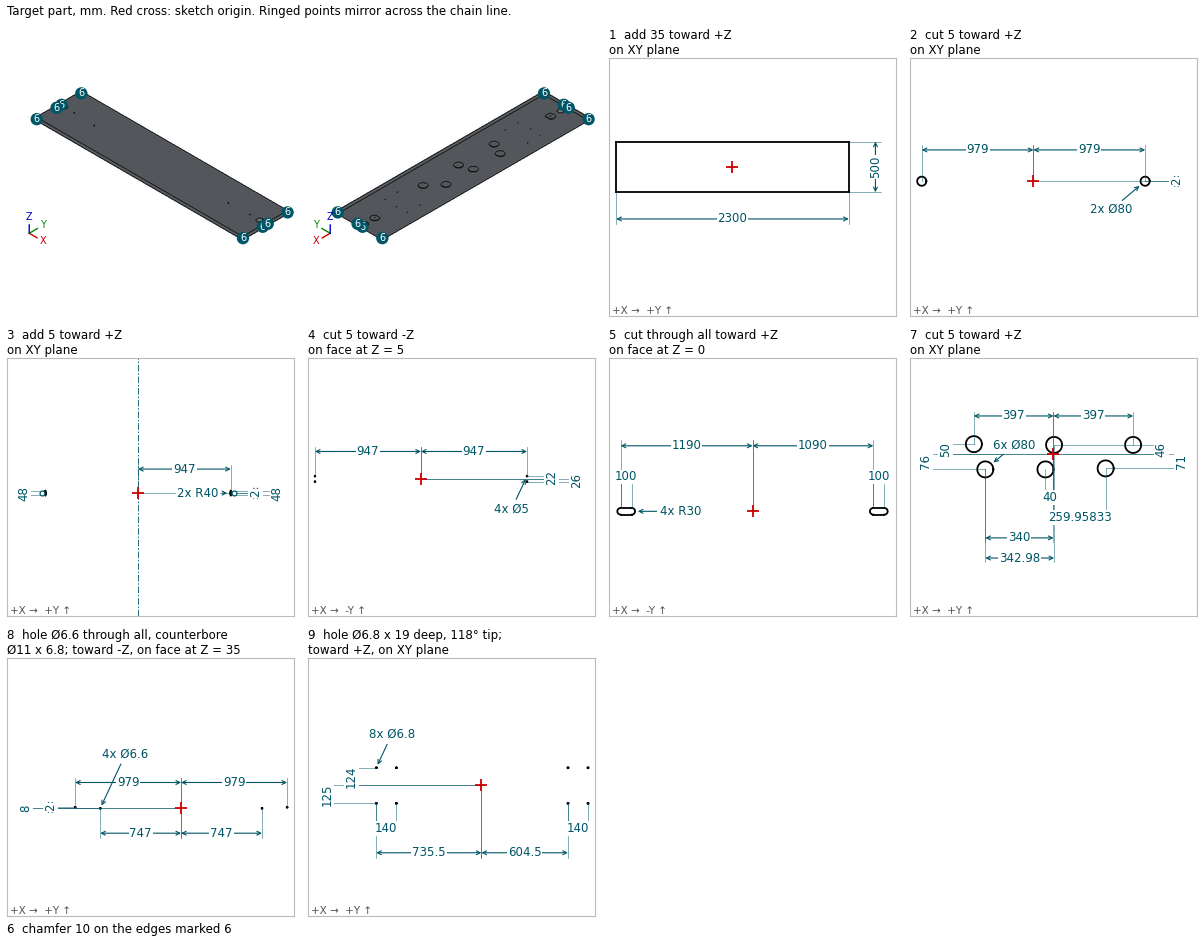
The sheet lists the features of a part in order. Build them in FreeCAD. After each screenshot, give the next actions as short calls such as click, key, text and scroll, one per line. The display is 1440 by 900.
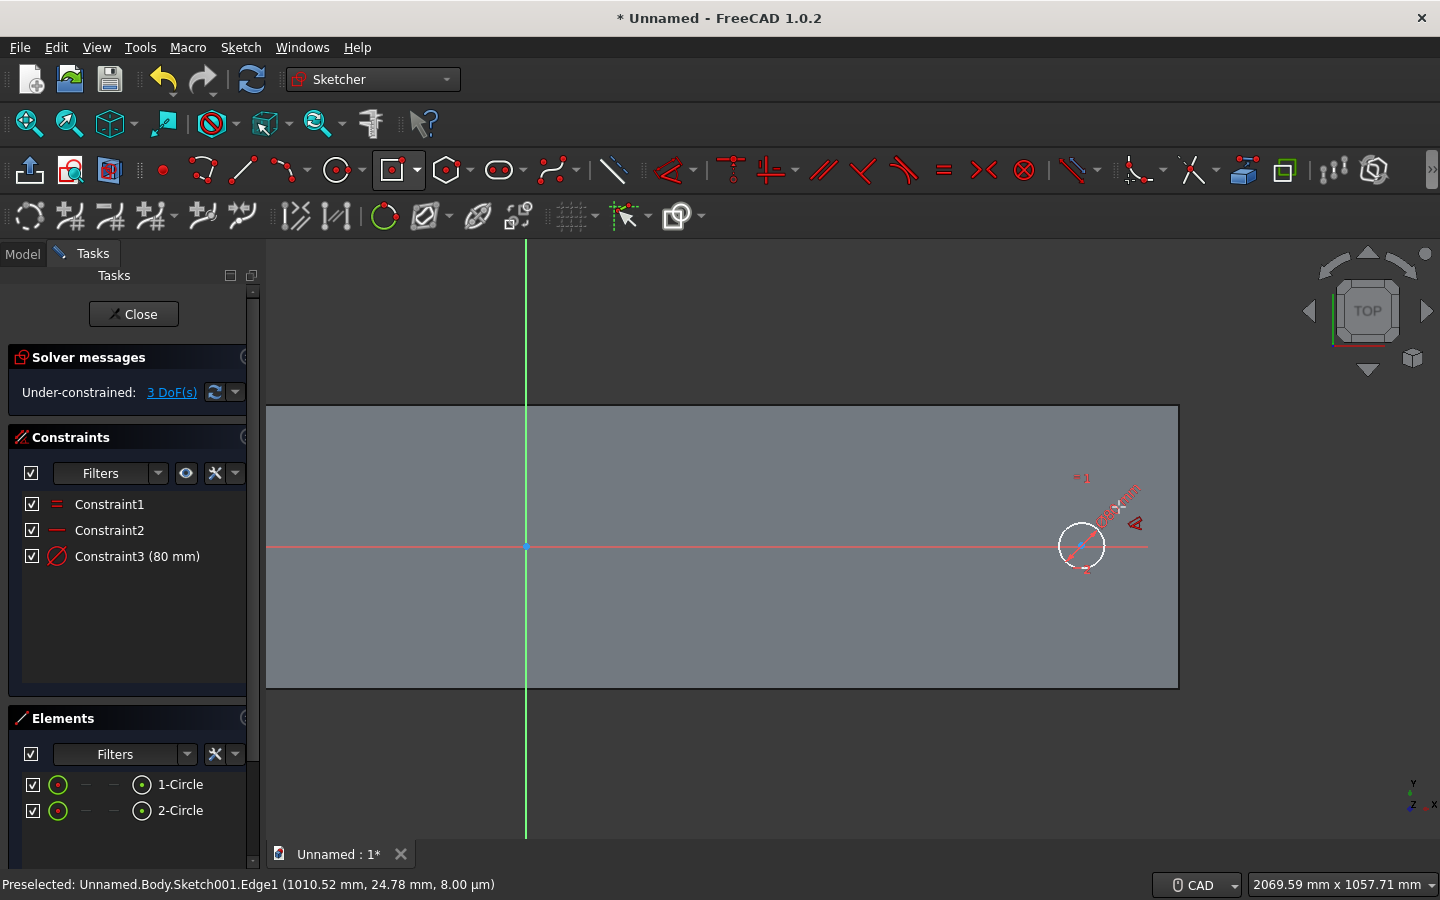
scroll(1082, 546, up, 18)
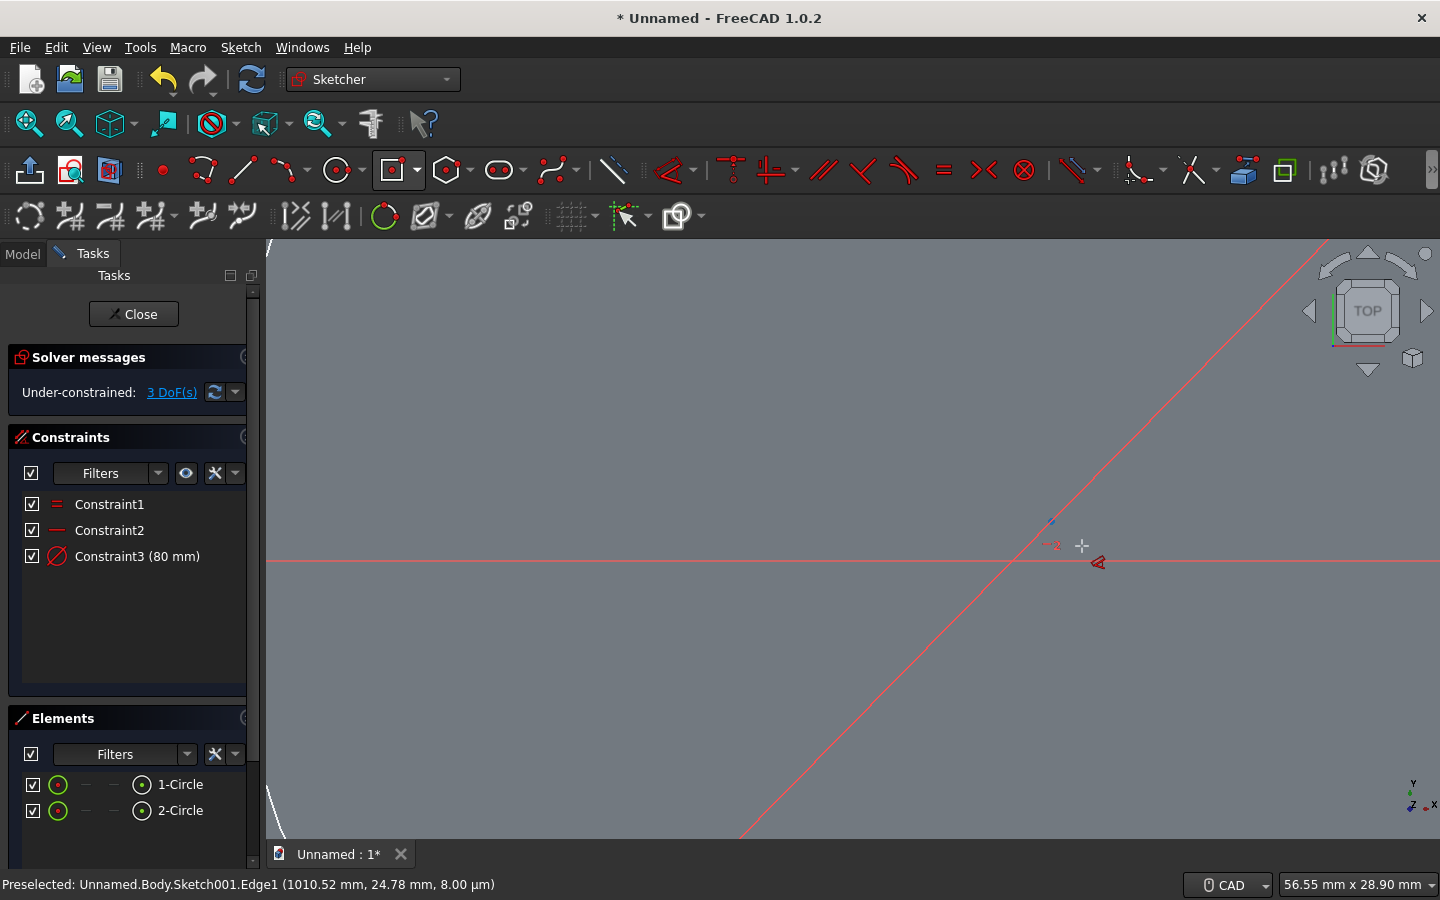
click(1052, 521)
click(1086, 541)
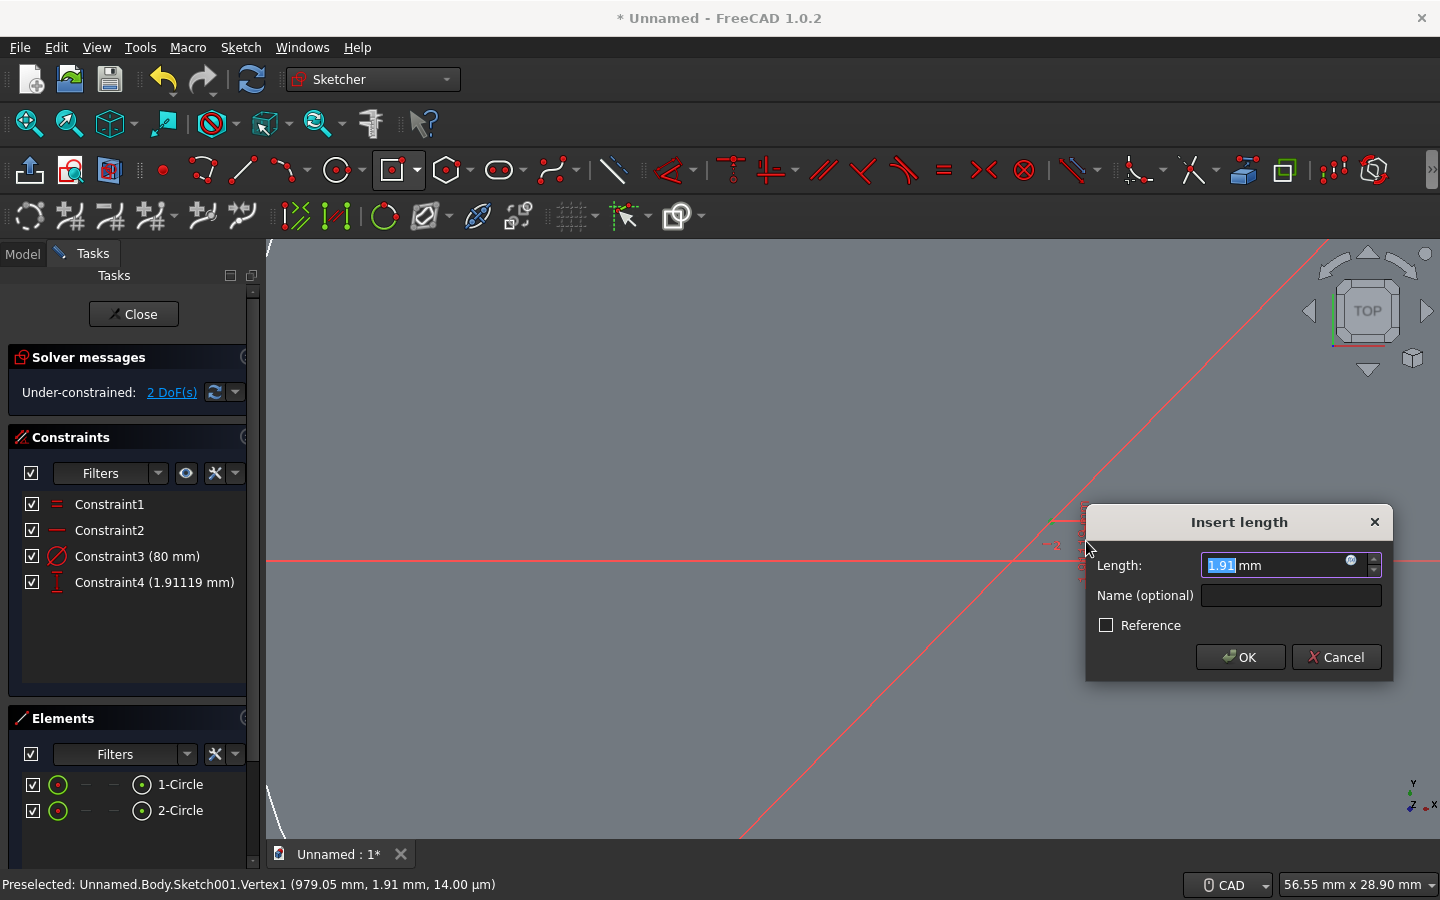
text(2)
key(Return)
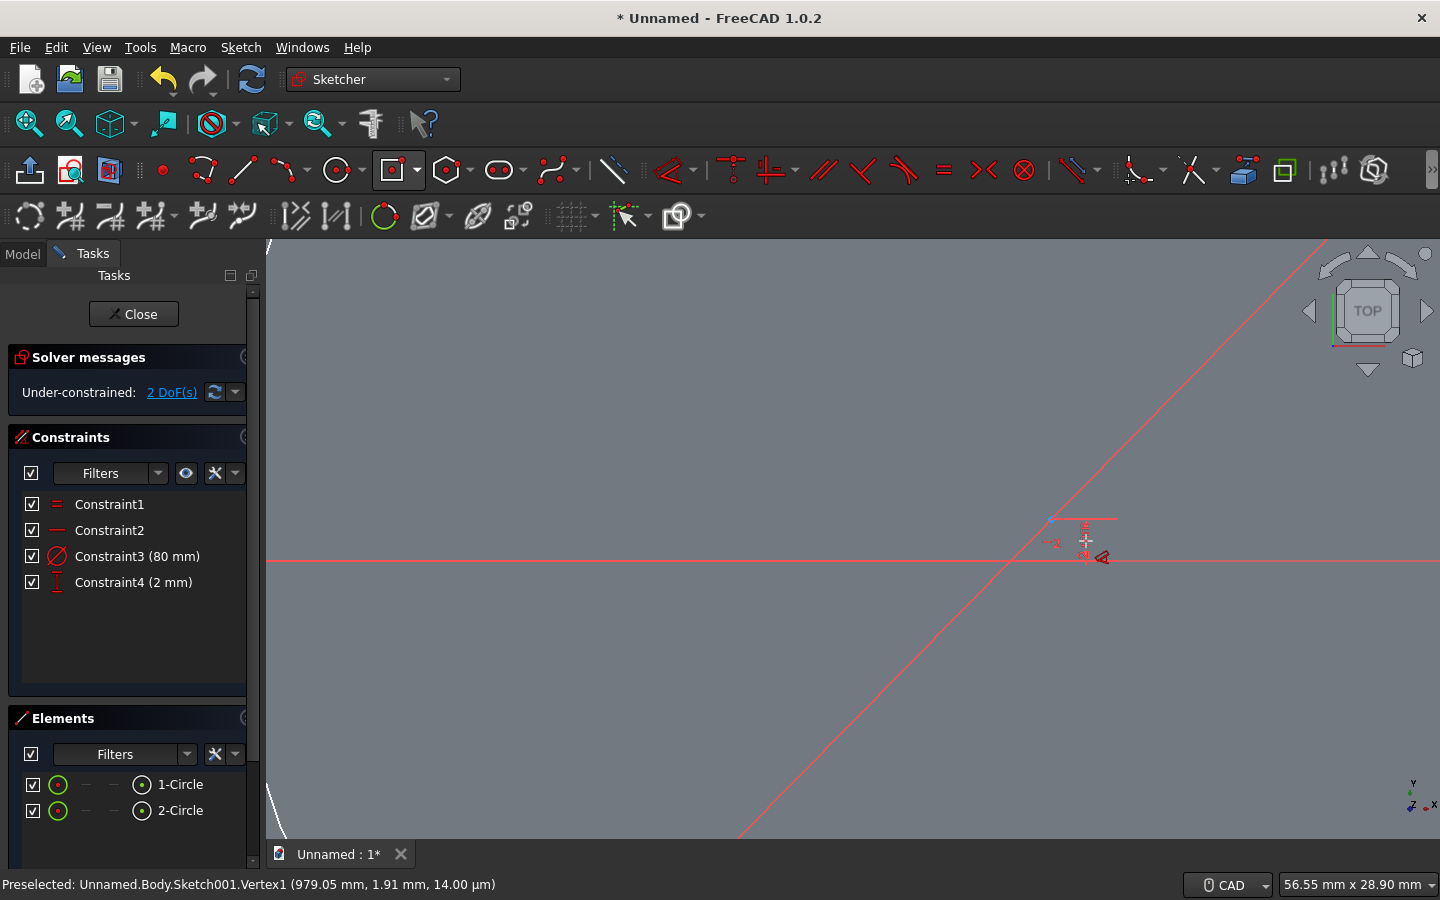
scroll(784, 539, down, 15)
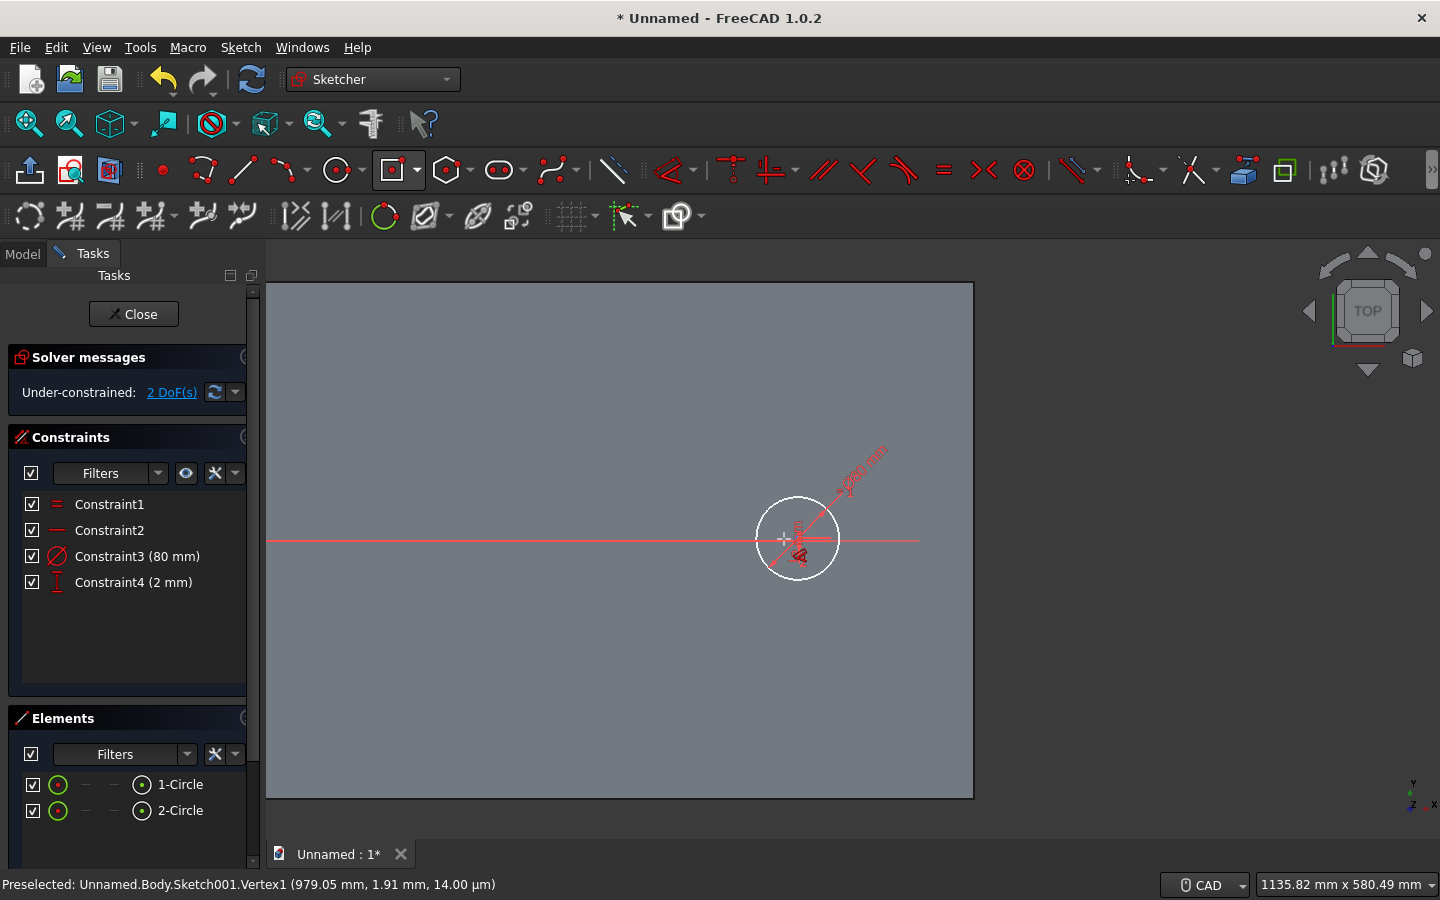
scroll(1215, 539, down, 6)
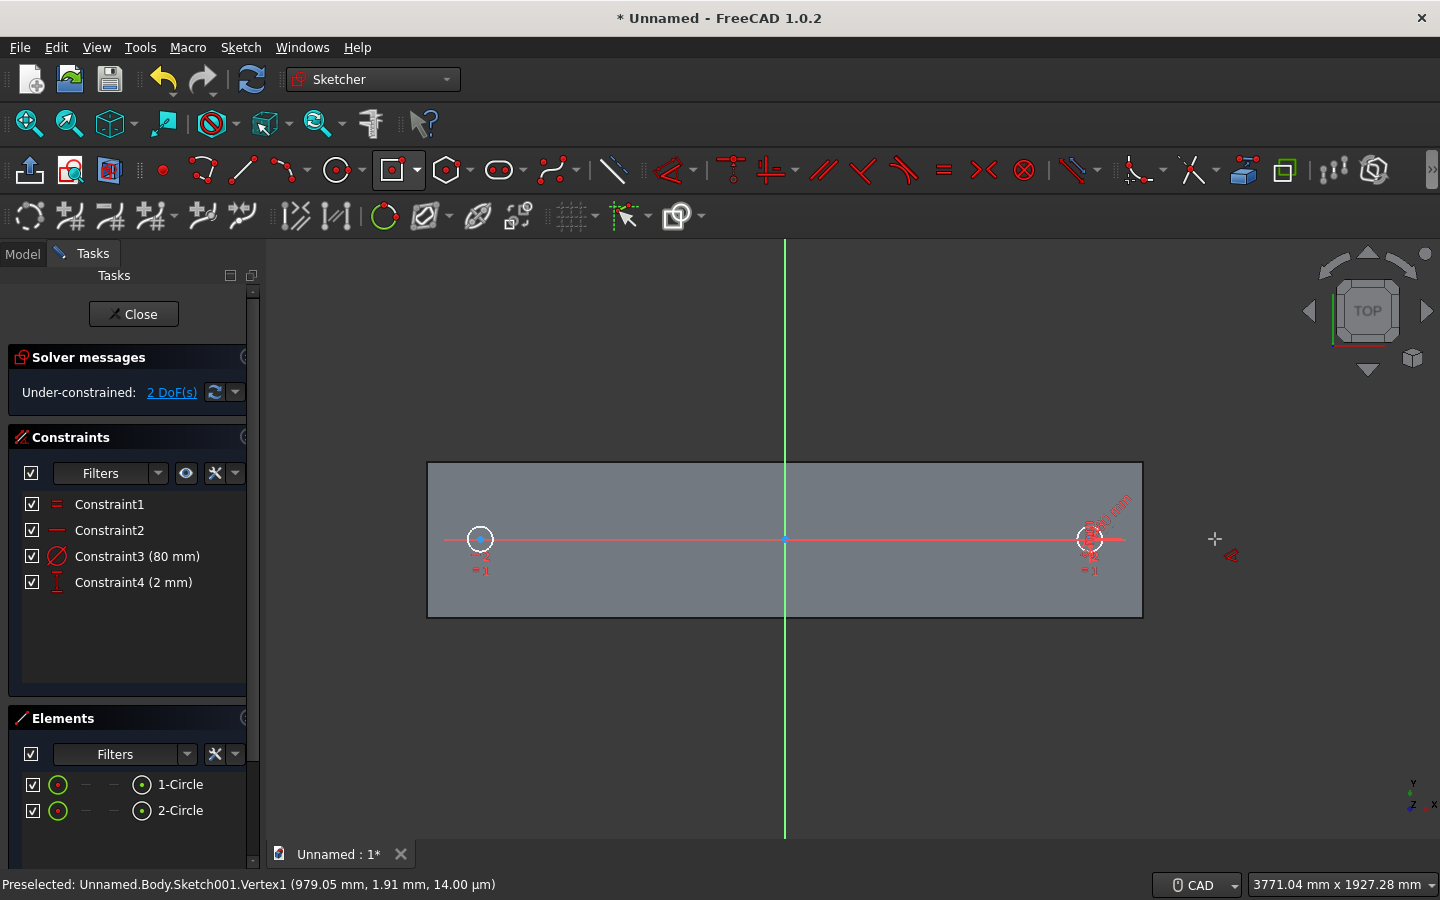
click(1090, 539)
click(937, 574)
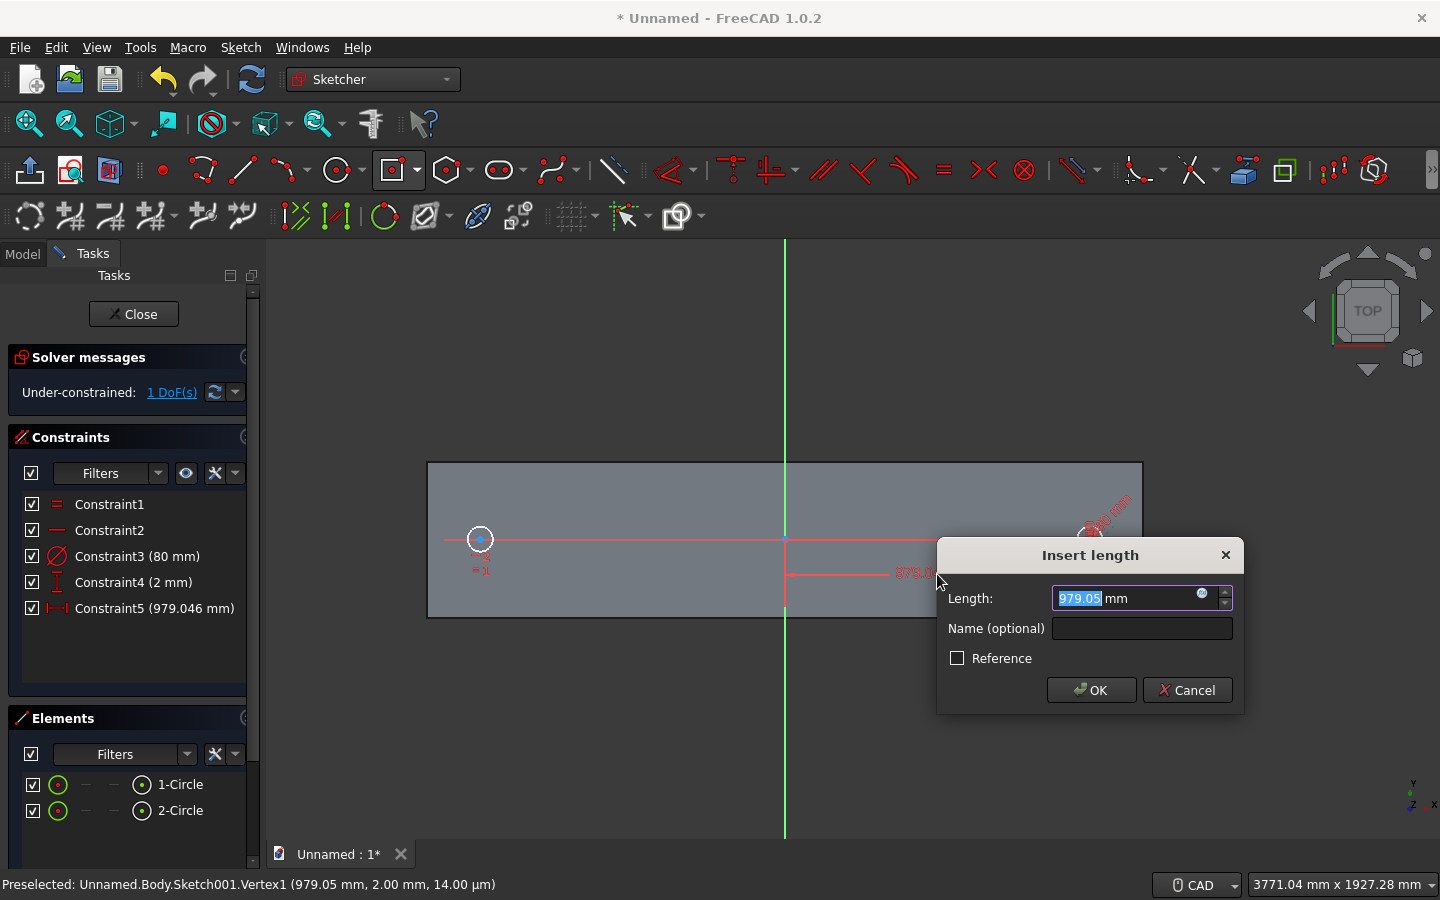
text(979)
key(Return)